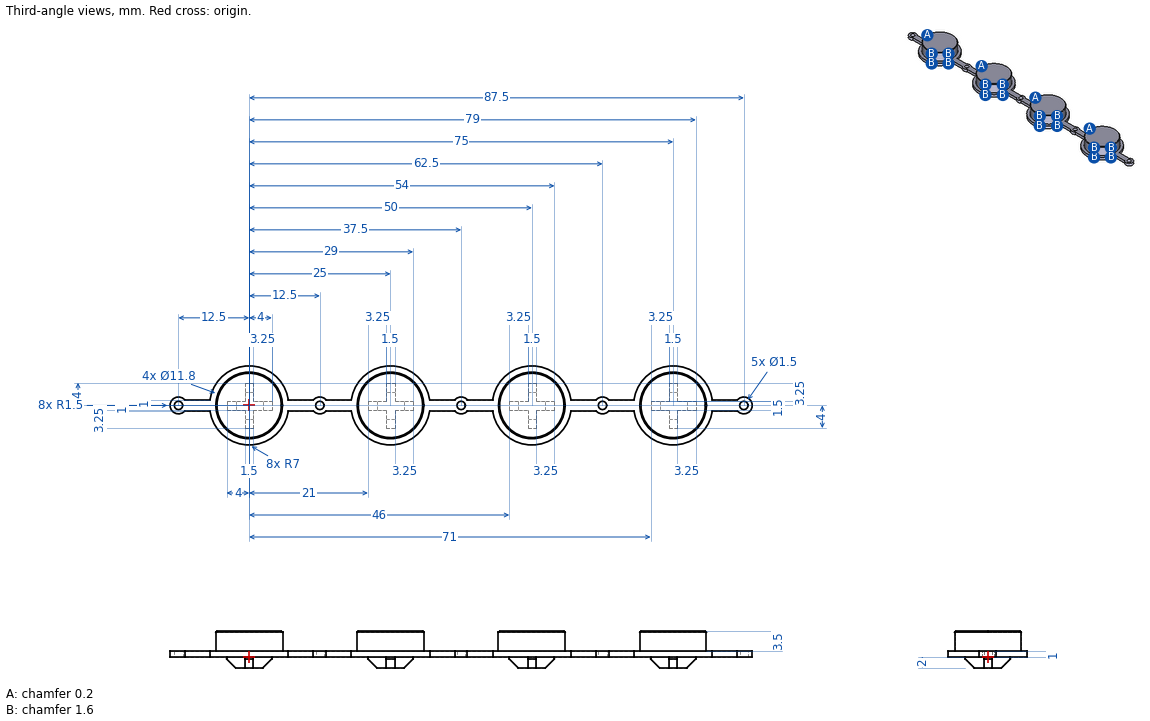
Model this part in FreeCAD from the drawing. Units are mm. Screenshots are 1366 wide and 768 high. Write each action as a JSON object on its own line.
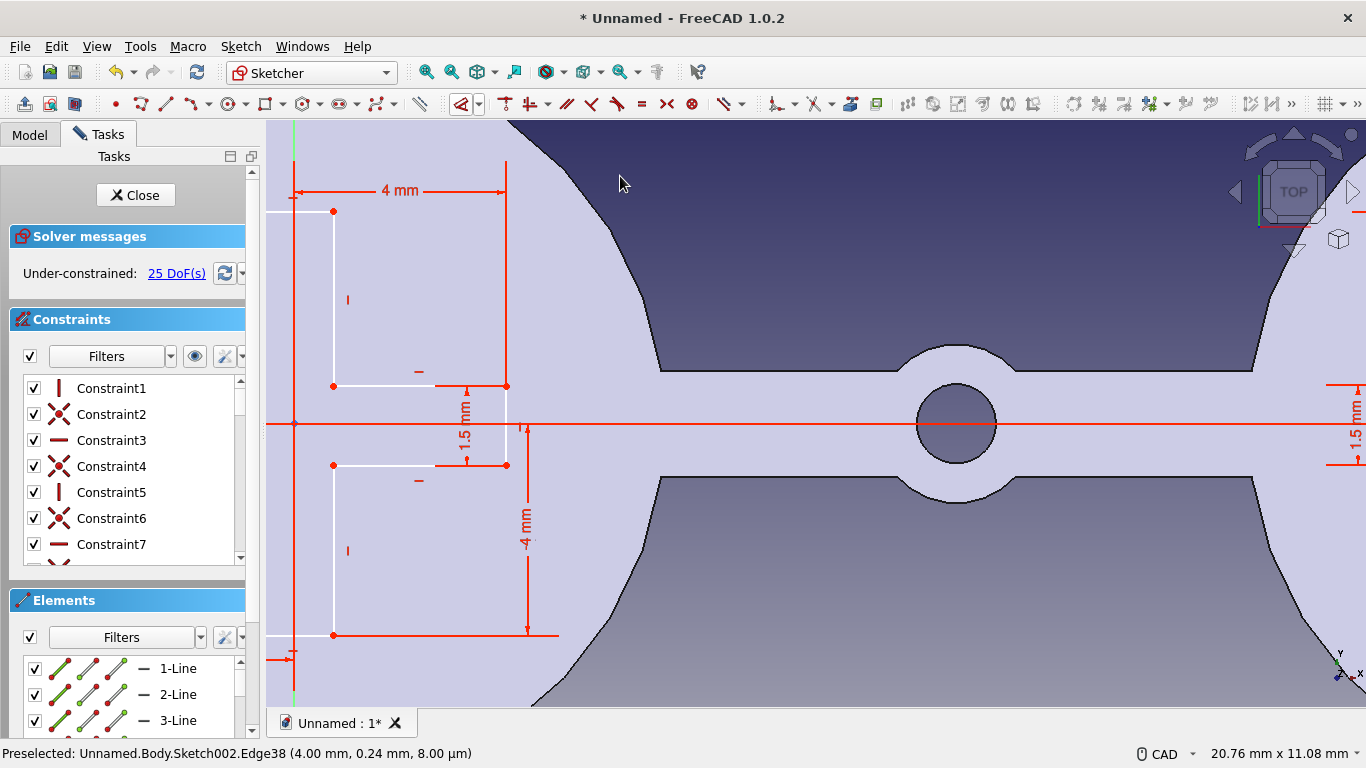
{"action": "left_click", "coordinate": [310, 636]}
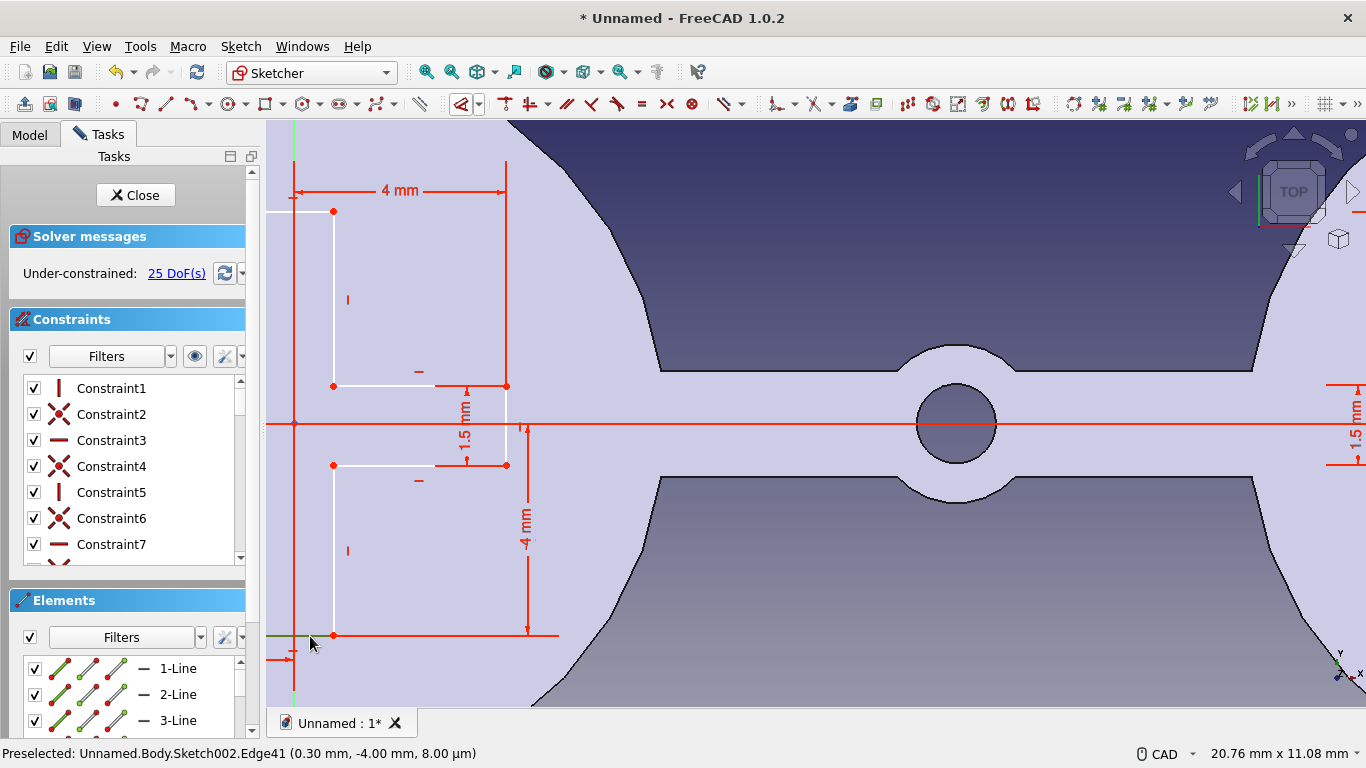
{"action": "key", "text": "l"}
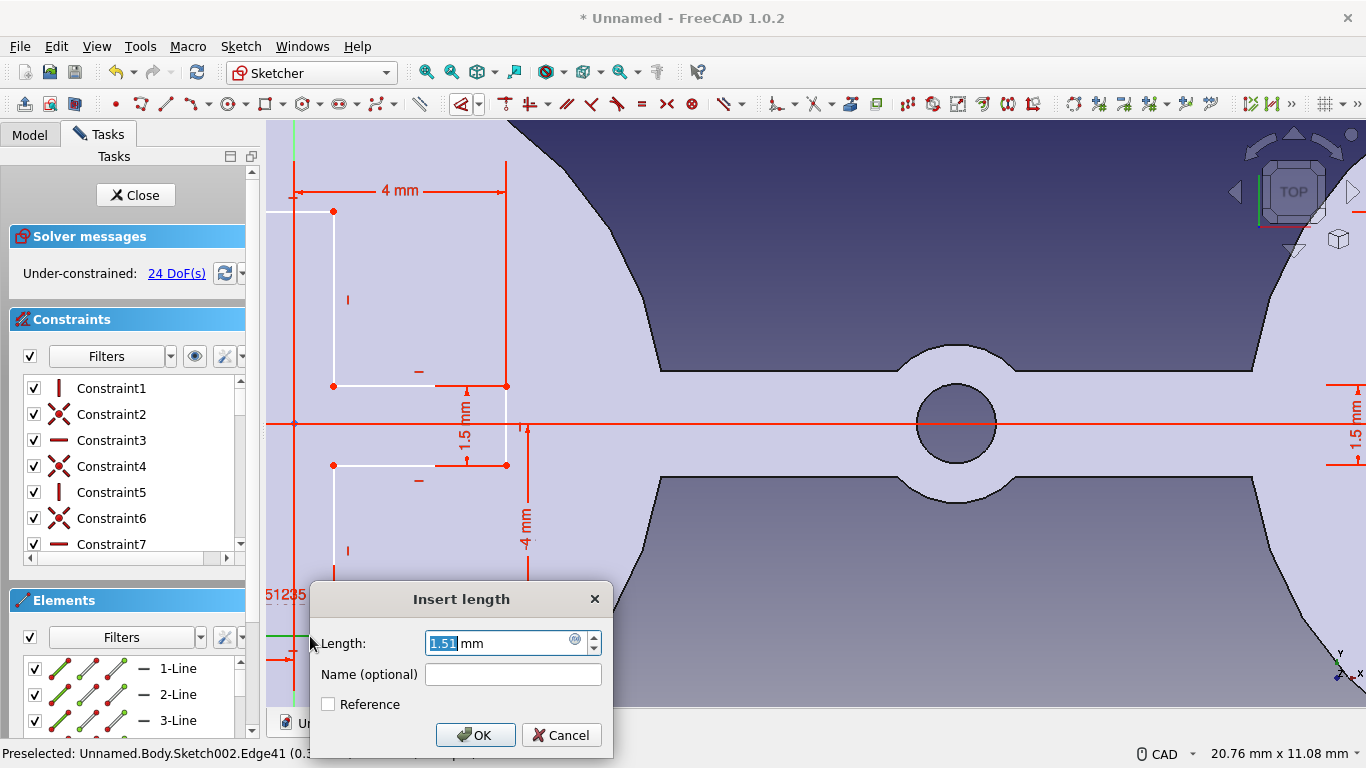
{"action": "type", "text": "1.5"}
{"action": "key", "text": "Return"}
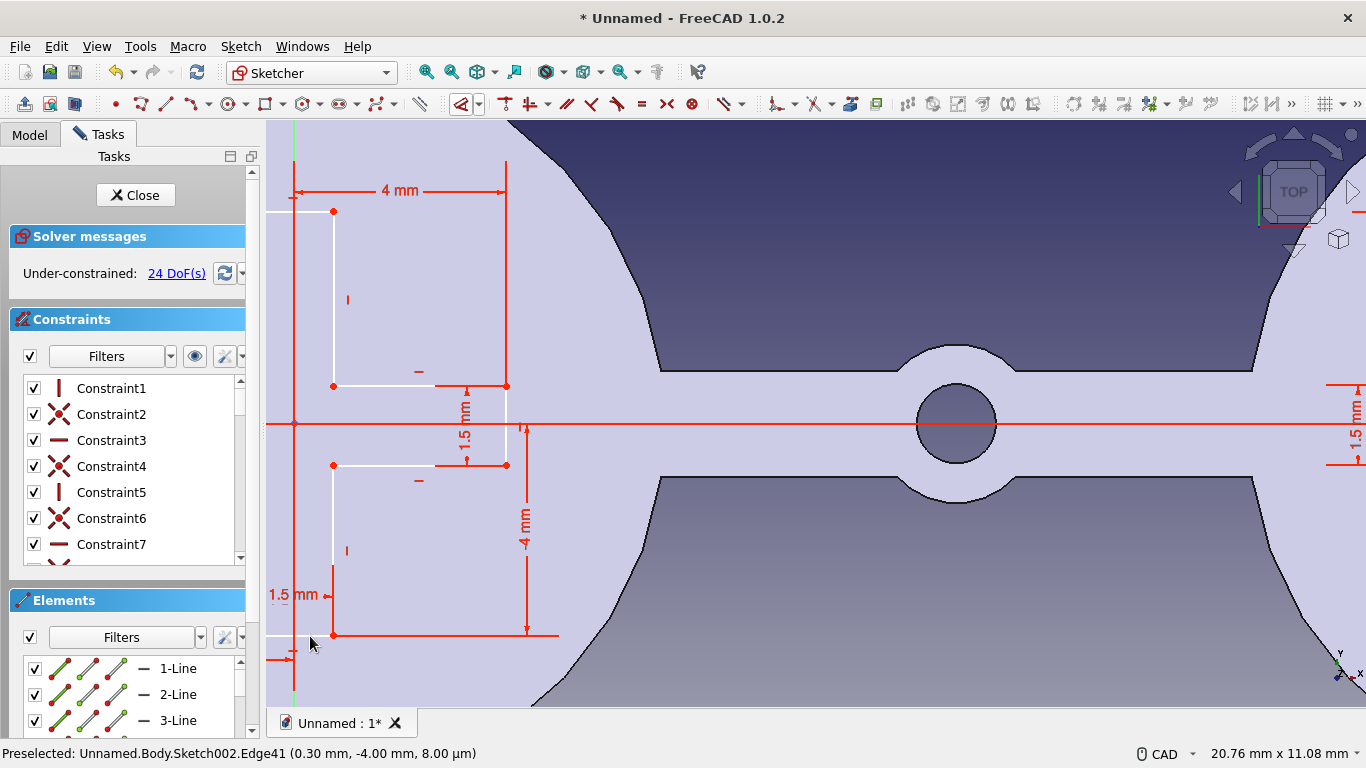
{"action": "scroll", "coordinate": [508, 412], "scroll_direction": "down", "scroll_amount": 10}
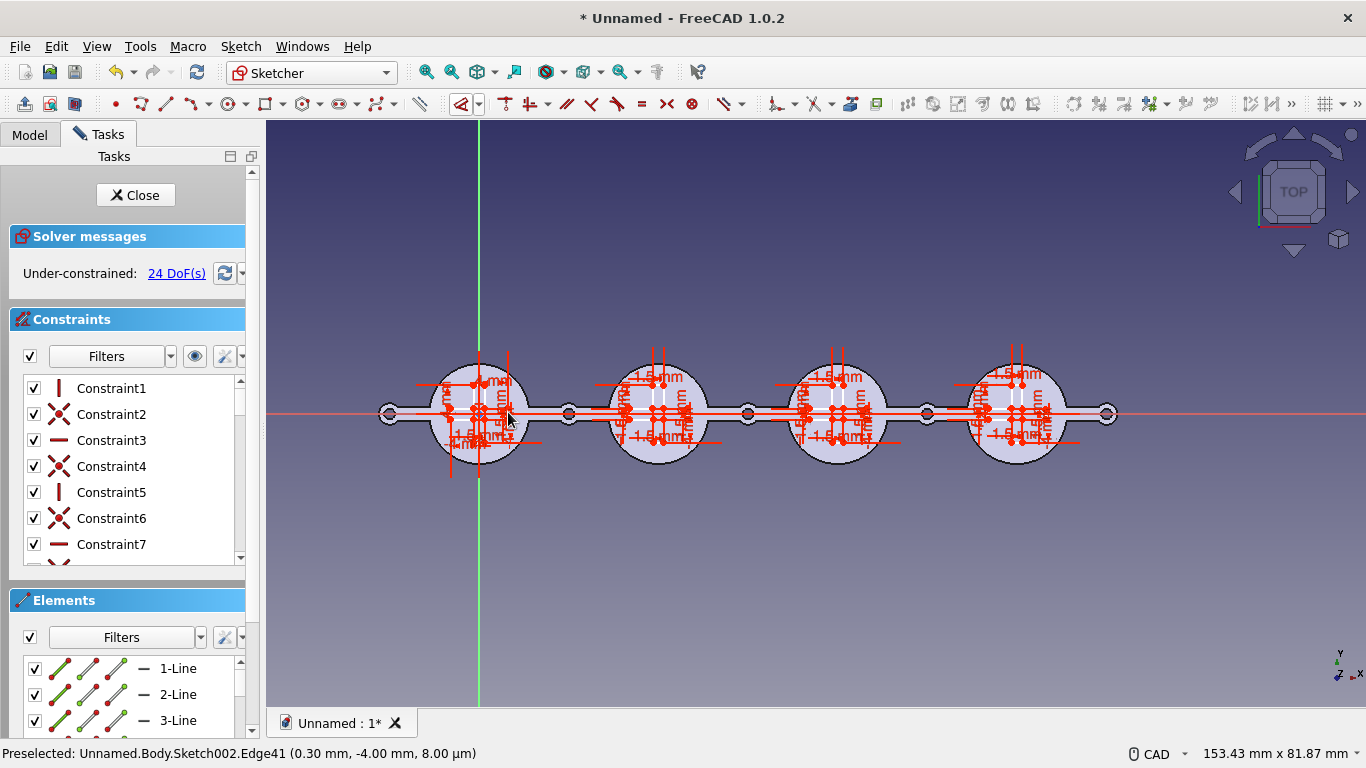
{"action": "scroll", "coordinate": [451, 416], "scroll_direction": "up", "scroll_amount": 9}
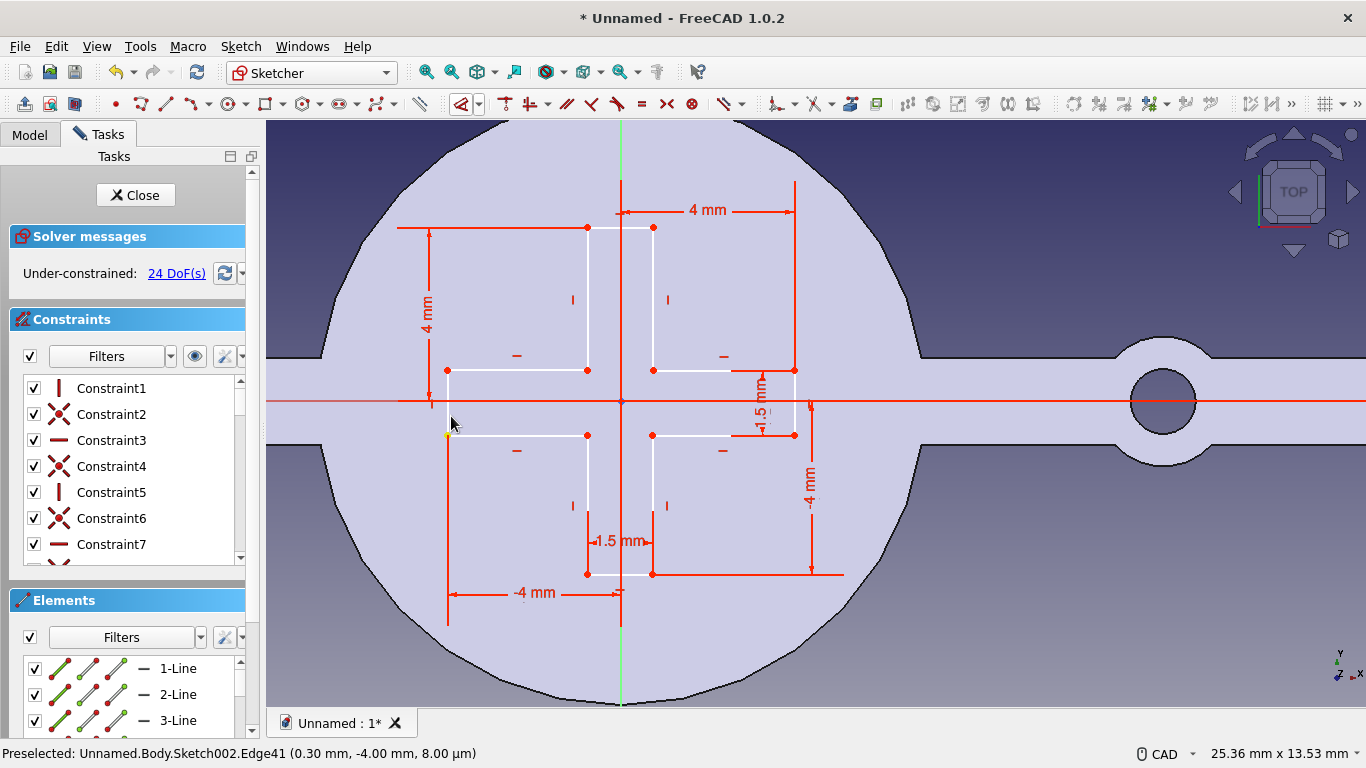
{"action": "left_click", "coordinate": [448, 416]}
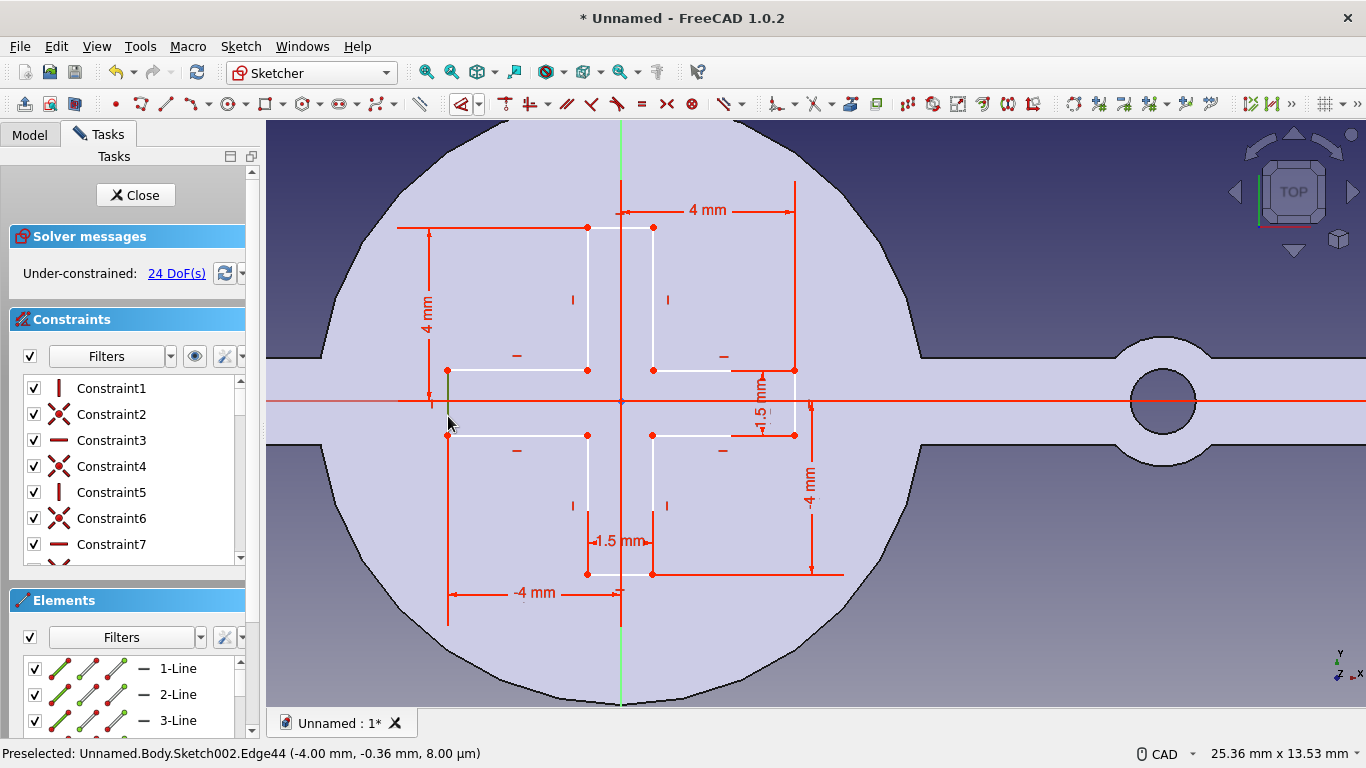
{"action": "key", "text": "i"}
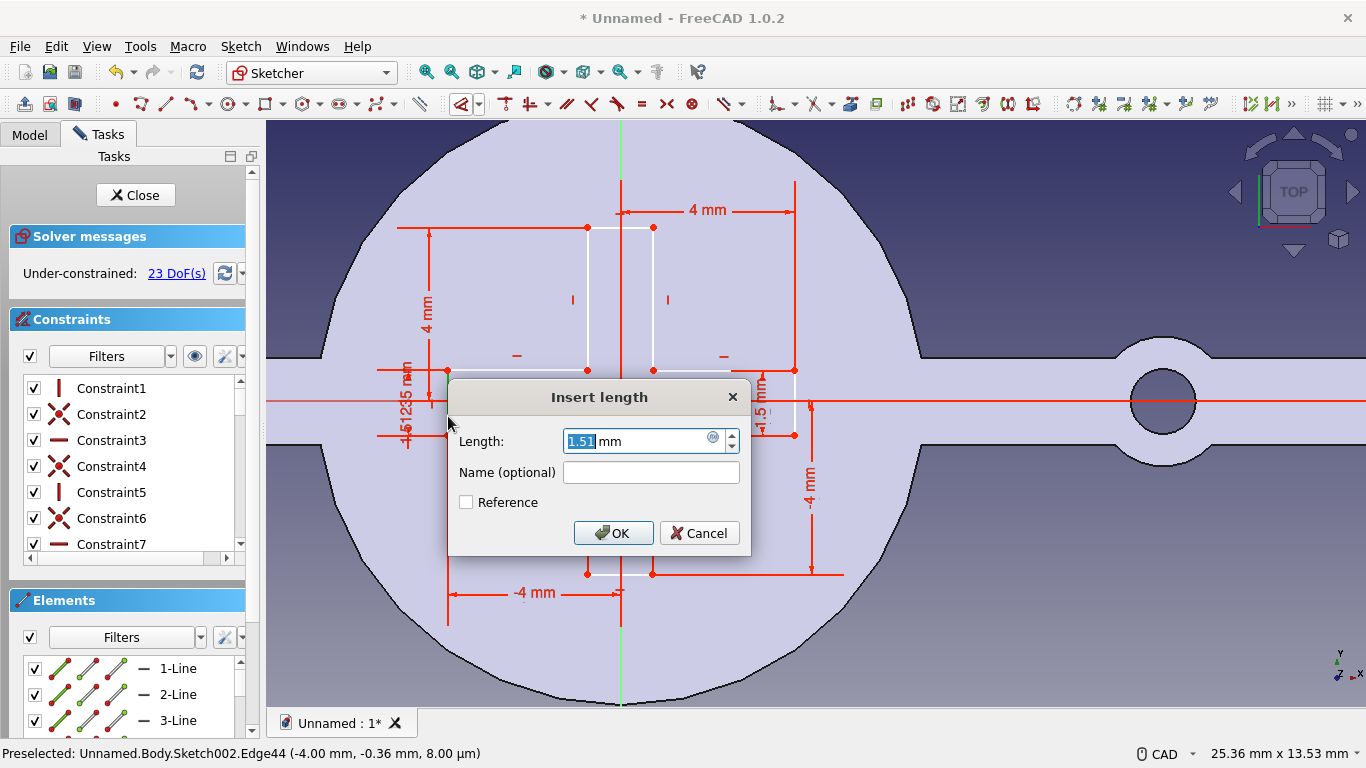
{"action": "type", "text": "1.5"}
{"action": "key", "text": "Return"}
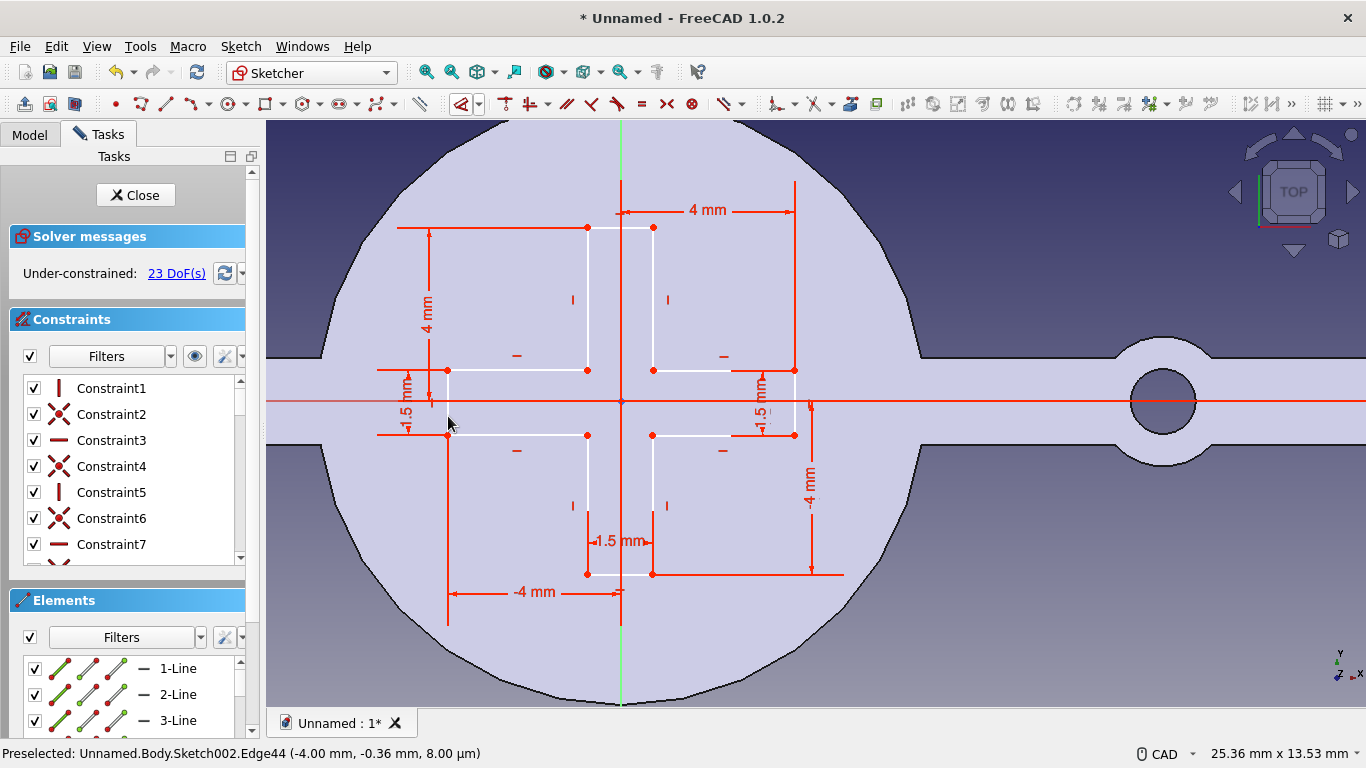
{"action": "left_click", "coordinate": [608, 228]}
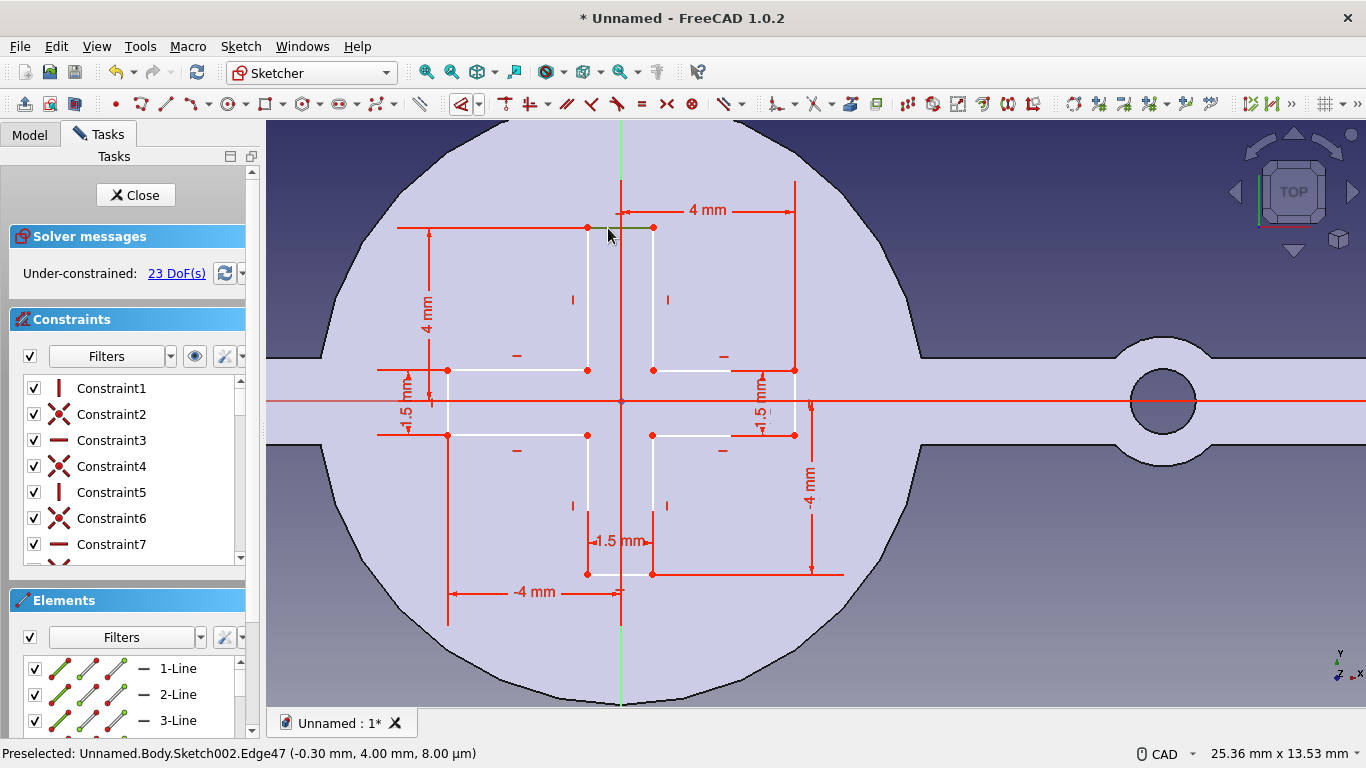
{"action": "key", "text": "l"}